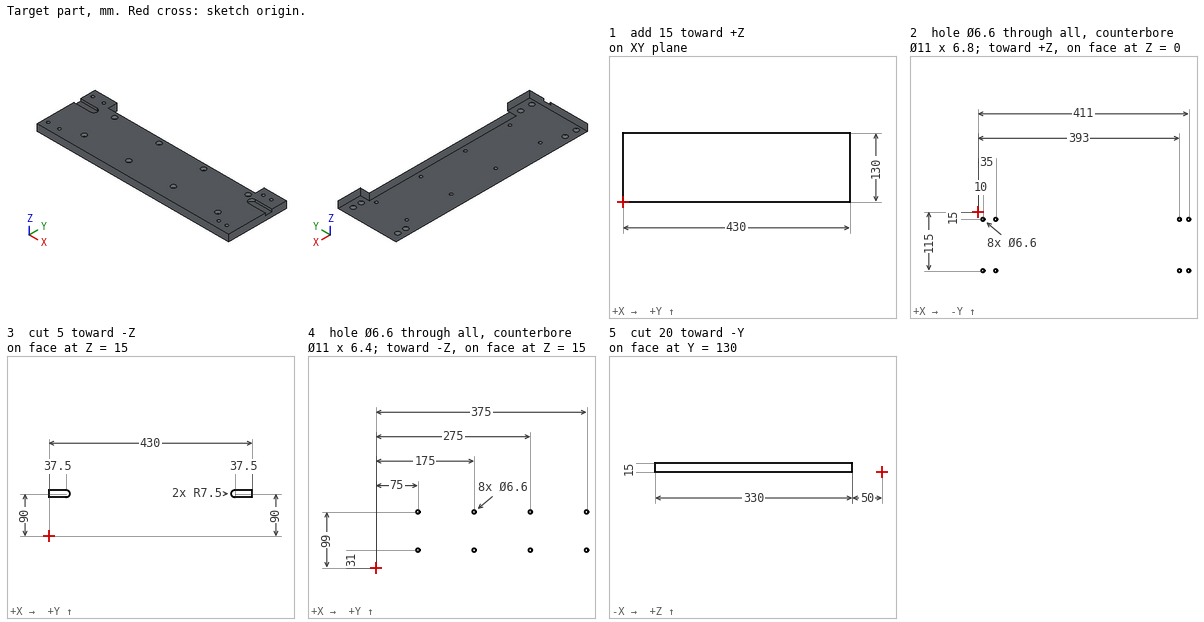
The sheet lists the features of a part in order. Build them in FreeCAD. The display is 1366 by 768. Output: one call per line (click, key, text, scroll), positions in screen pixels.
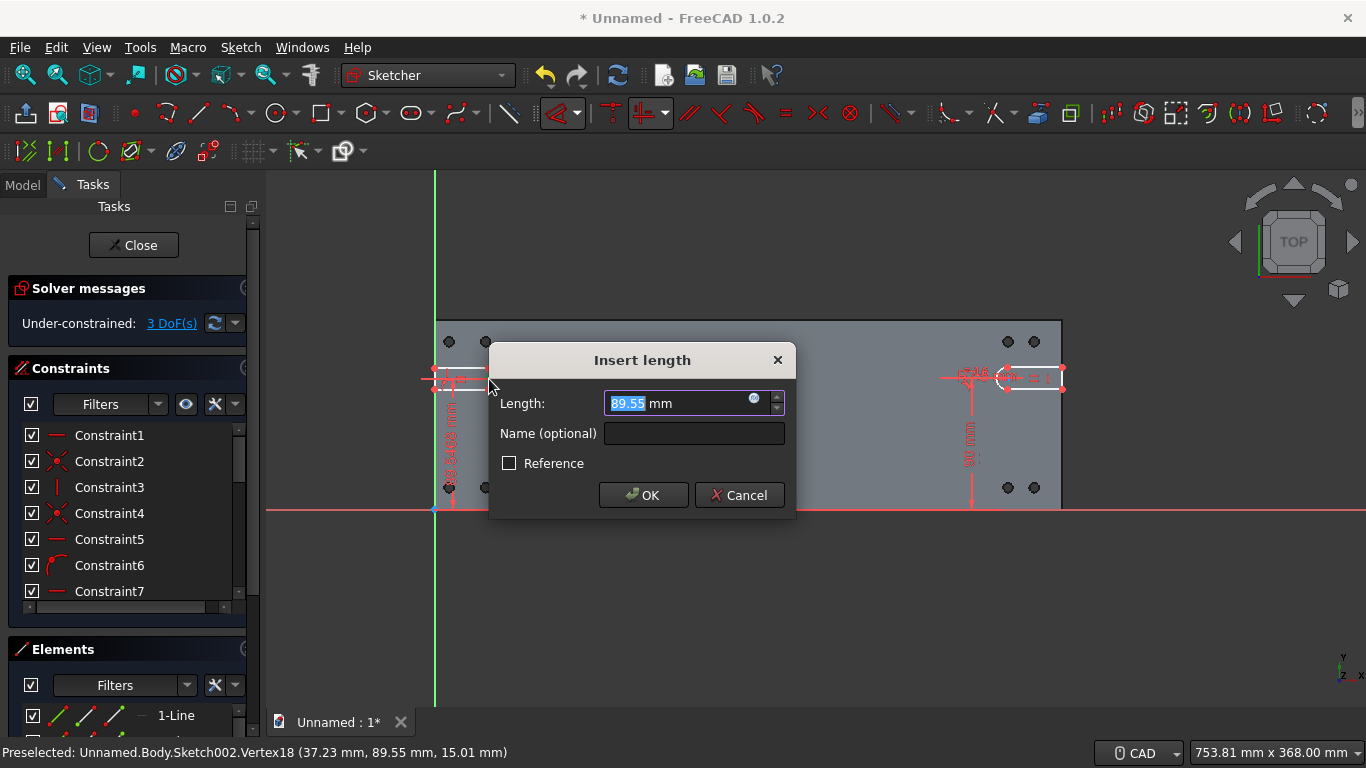
text(90)
key(Return)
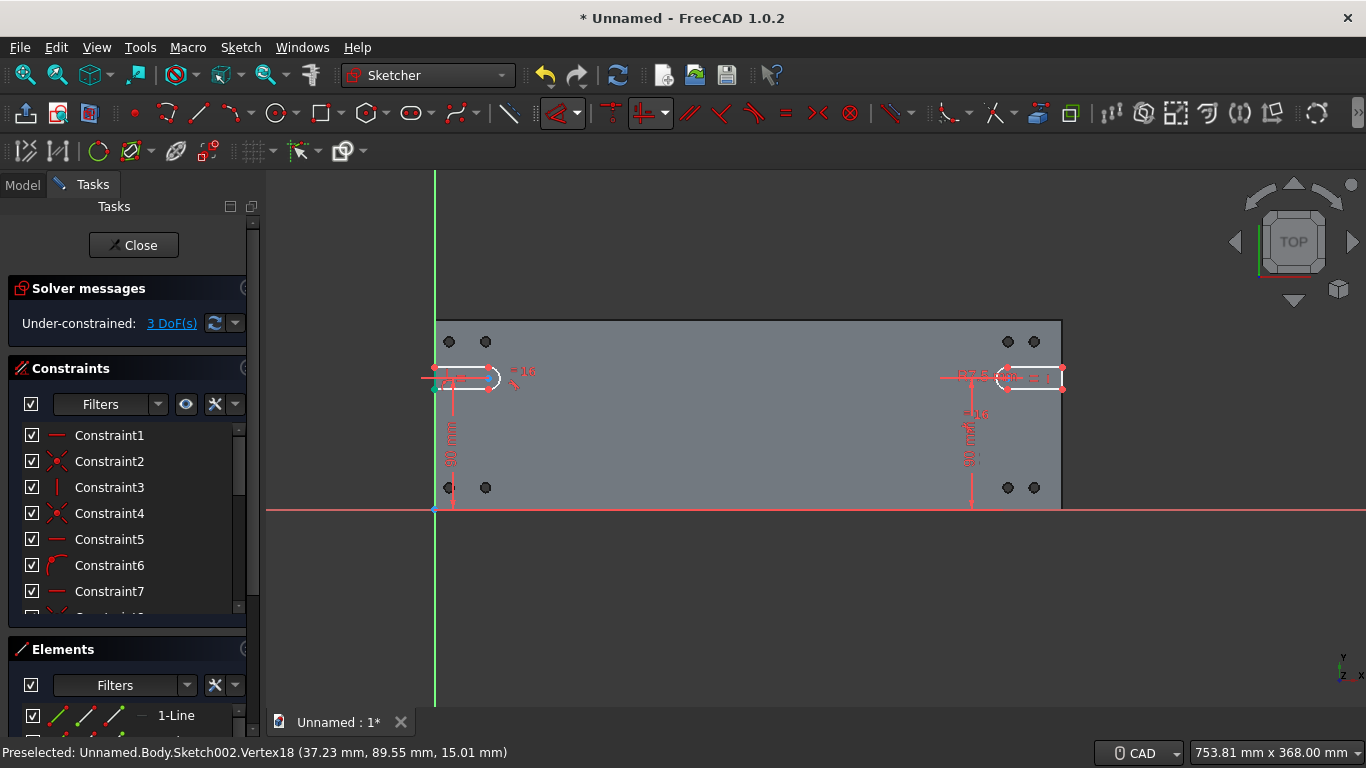
click(1024, 389)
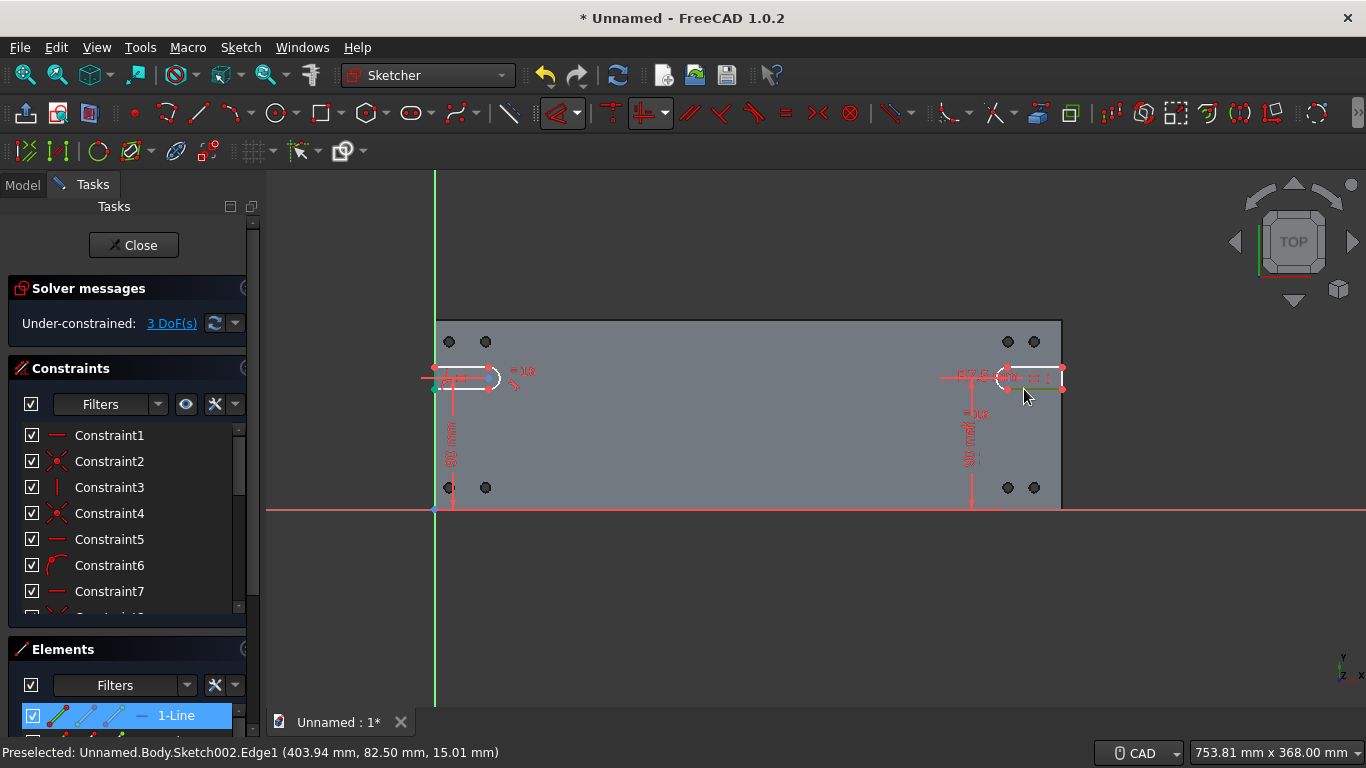
click(580, 114)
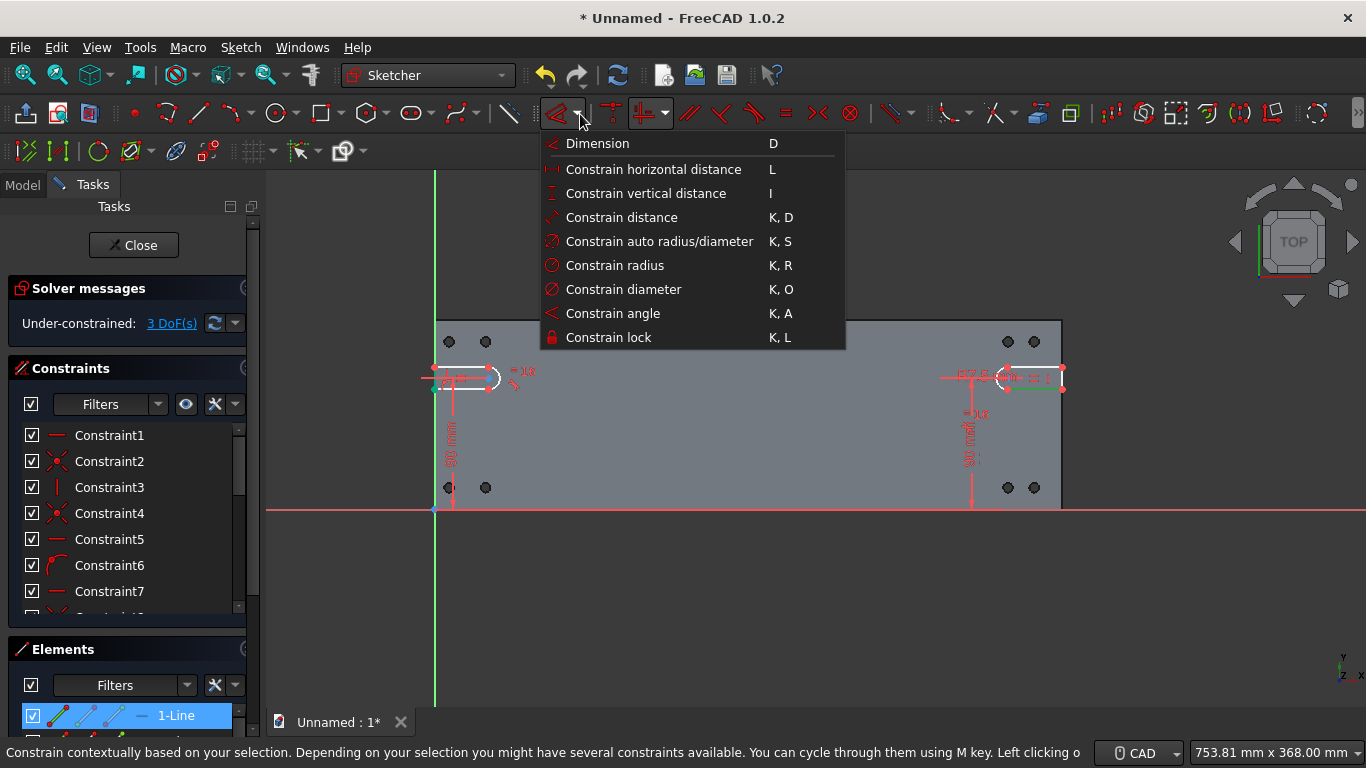
click(693, 169)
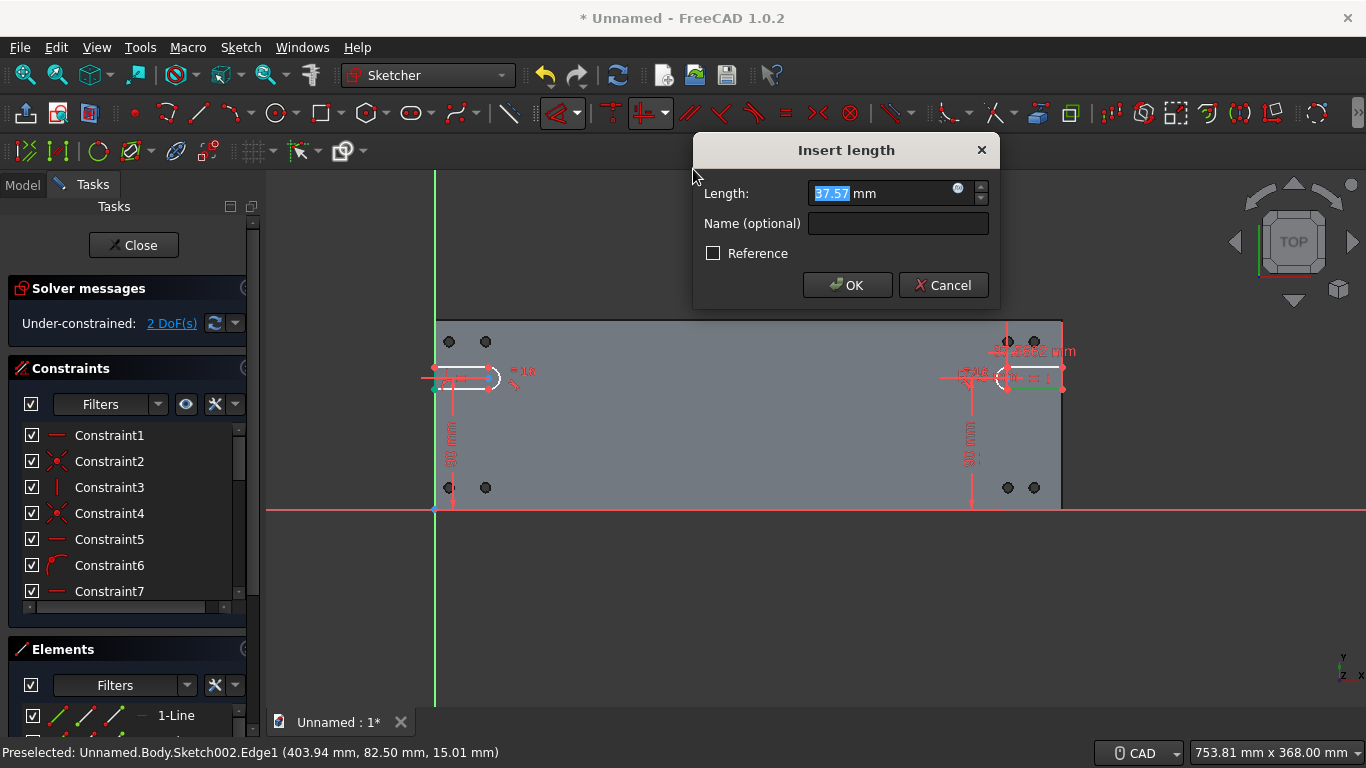
text(37.5)
key(Return)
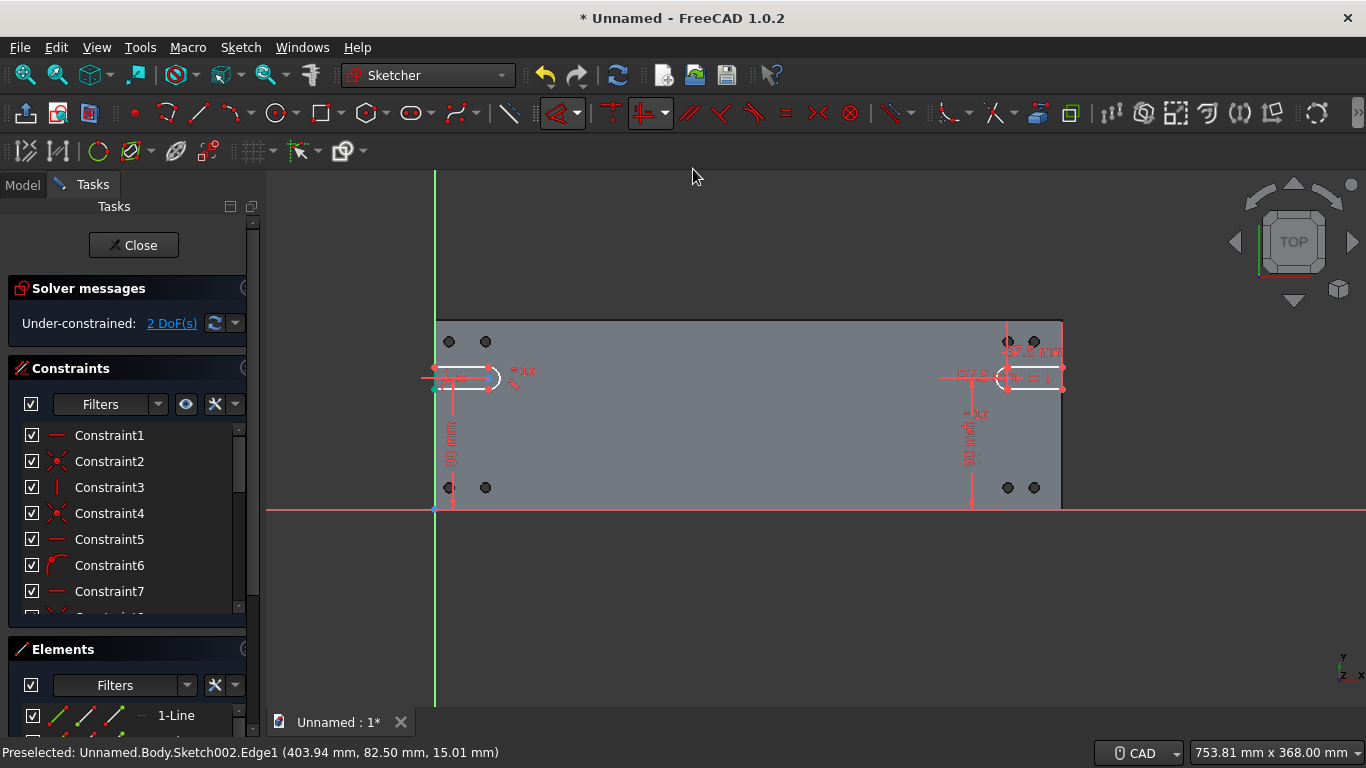
click(473, 367)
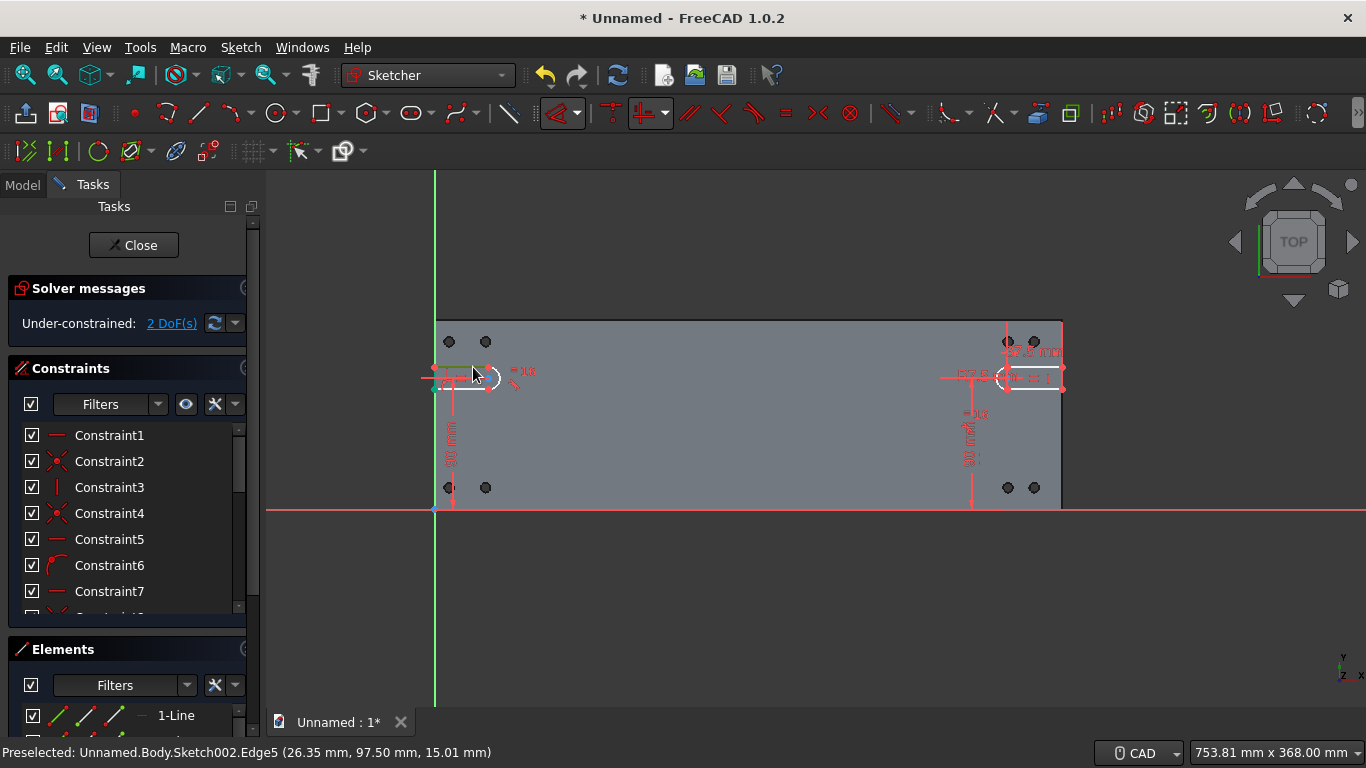
key(l)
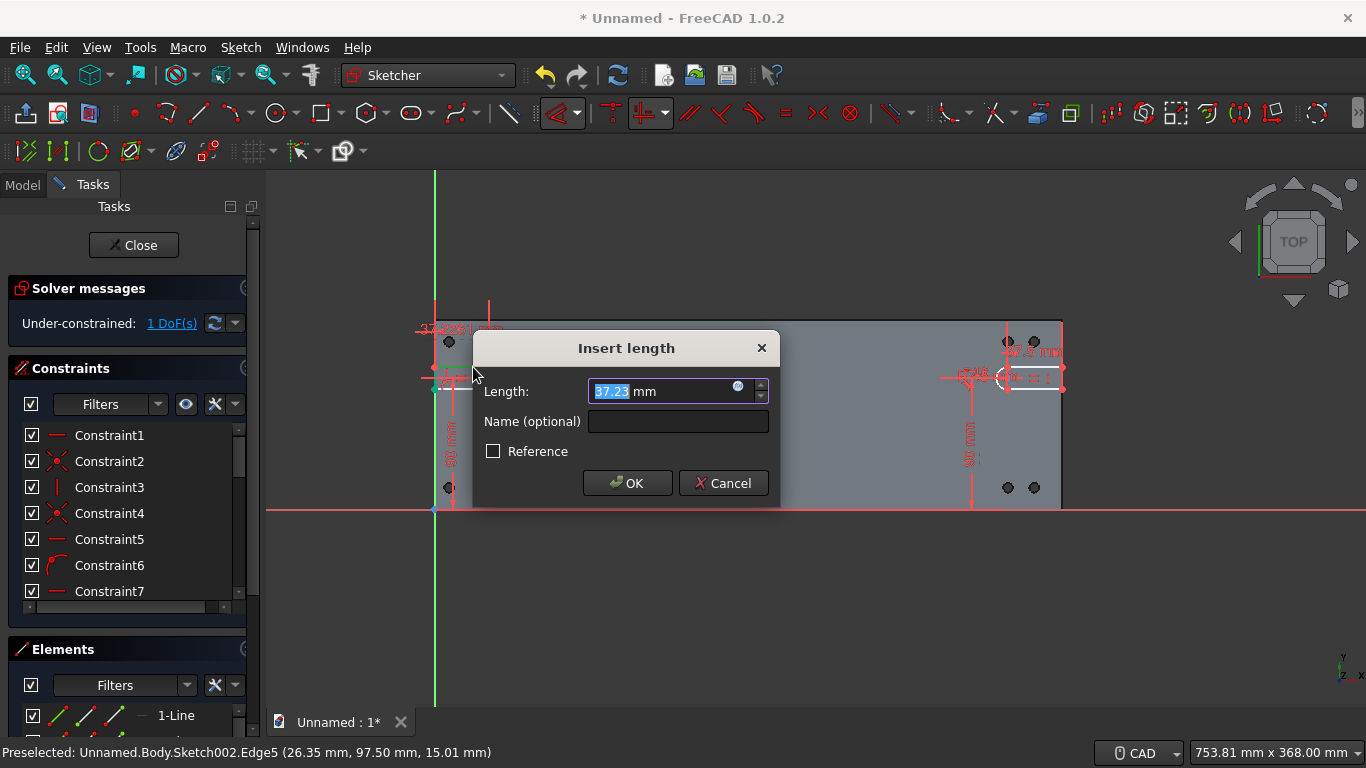
text(37.5)
key(Return)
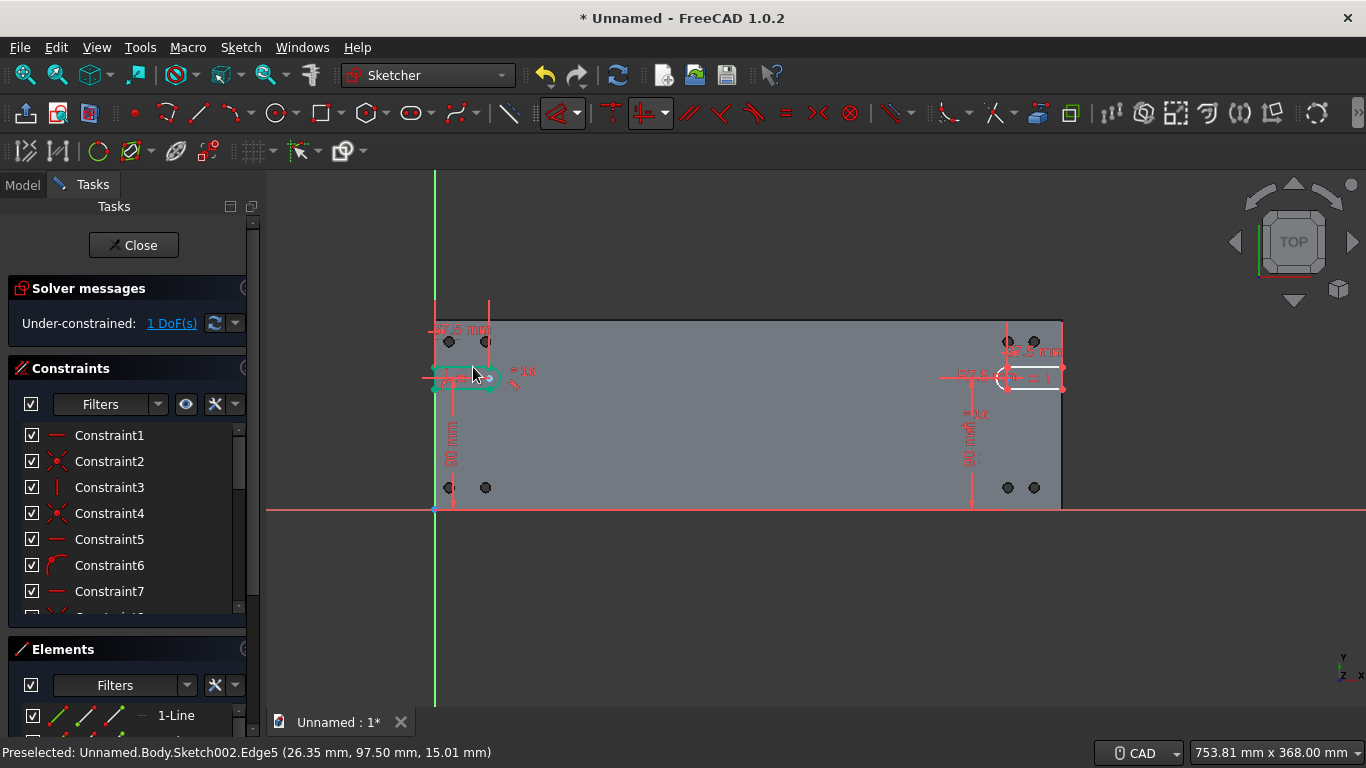
click(1062, 389)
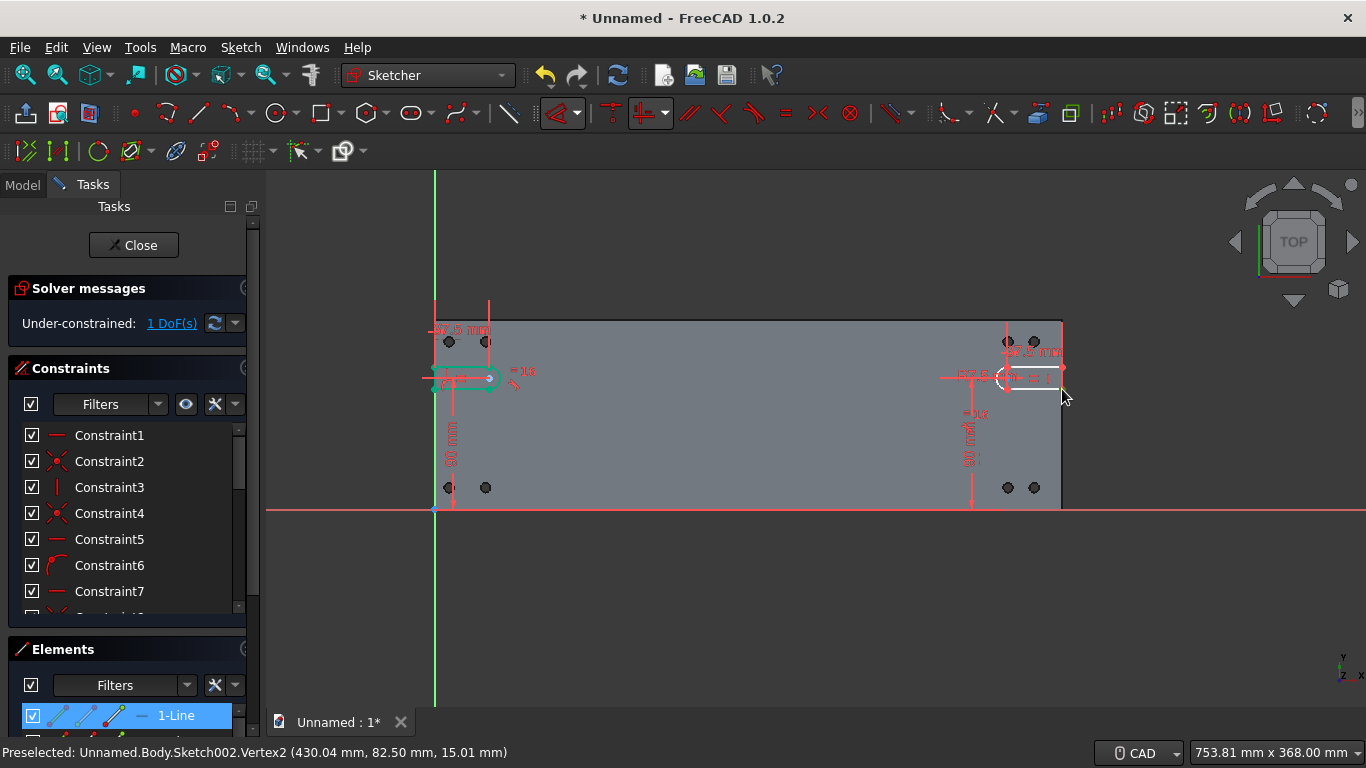
key(l)